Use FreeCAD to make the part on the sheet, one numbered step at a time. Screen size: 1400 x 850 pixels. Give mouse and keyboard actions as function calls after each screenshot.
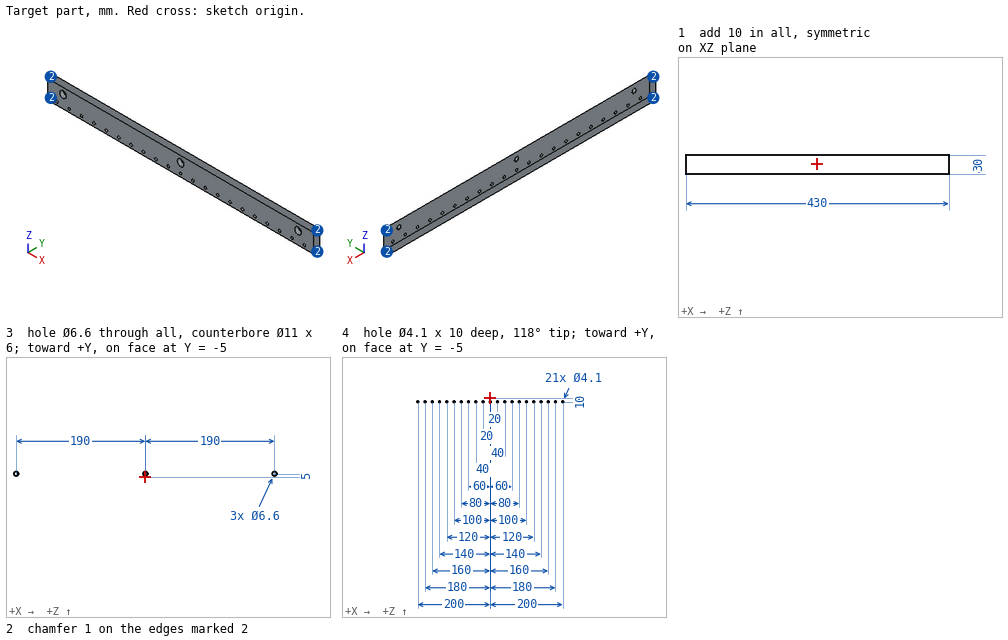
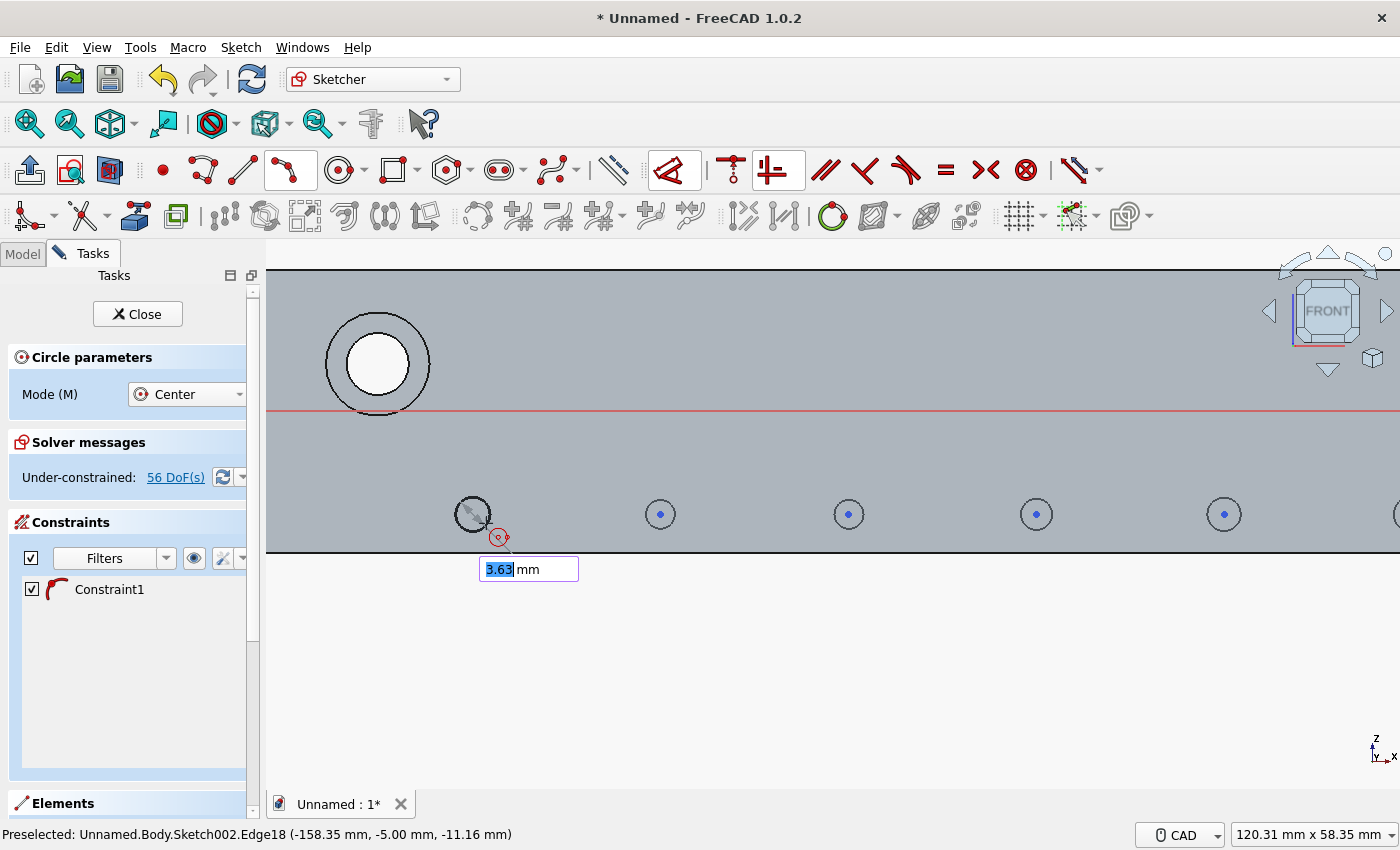
click(486, 519)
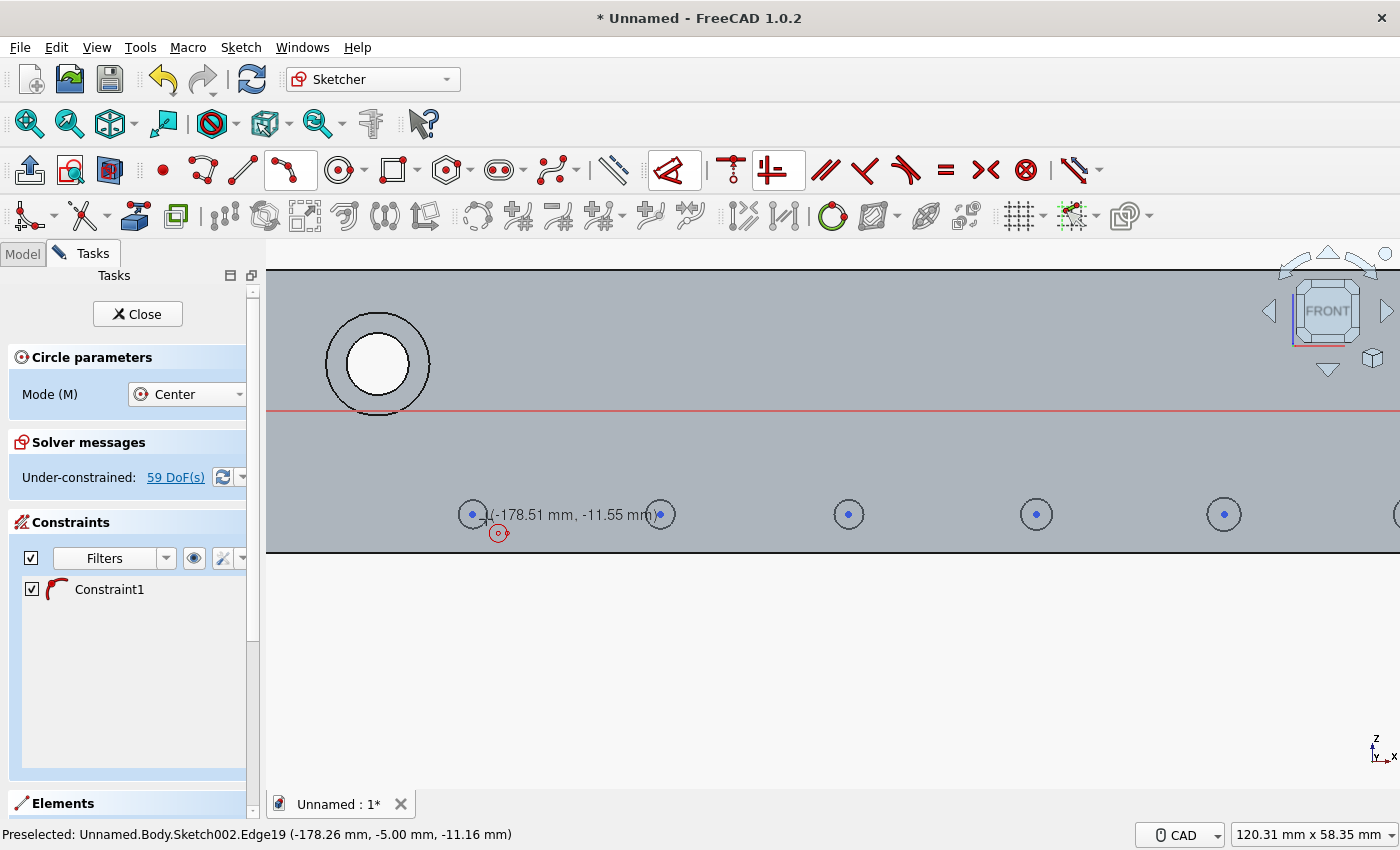
scroll(486, 523, down, 9)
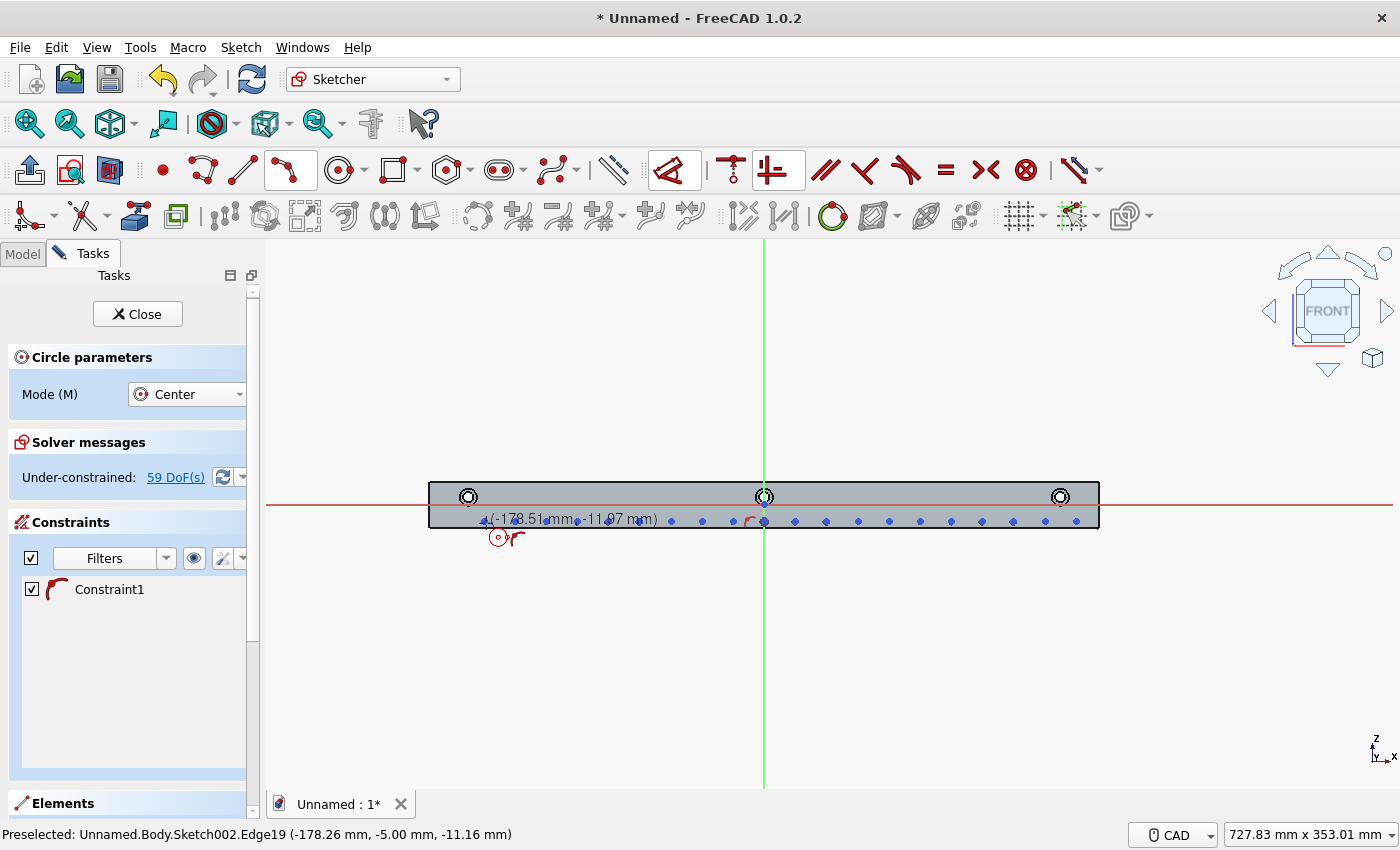
scroll(453, 521, up, 10)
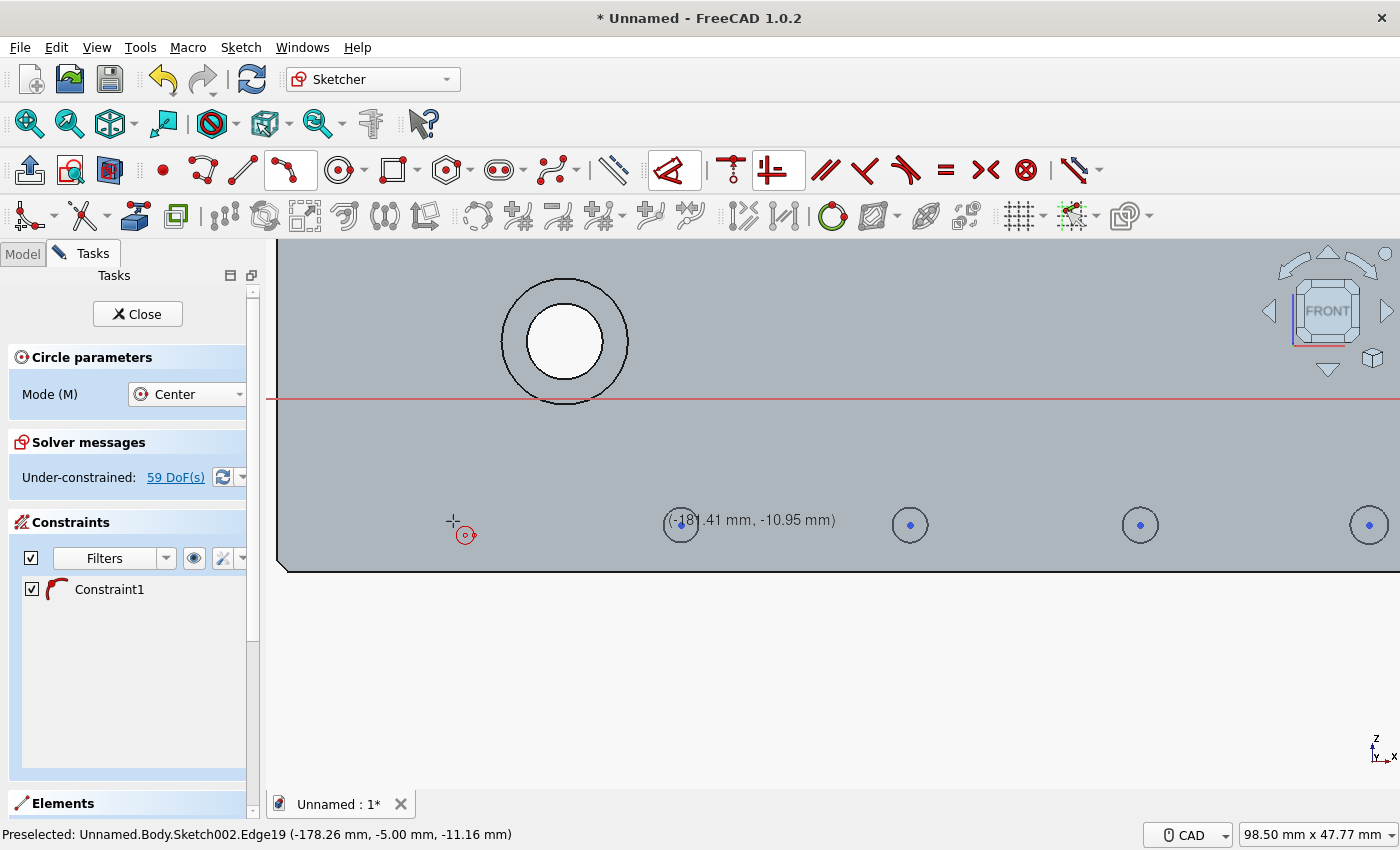
scroll(453, 521, down, 10)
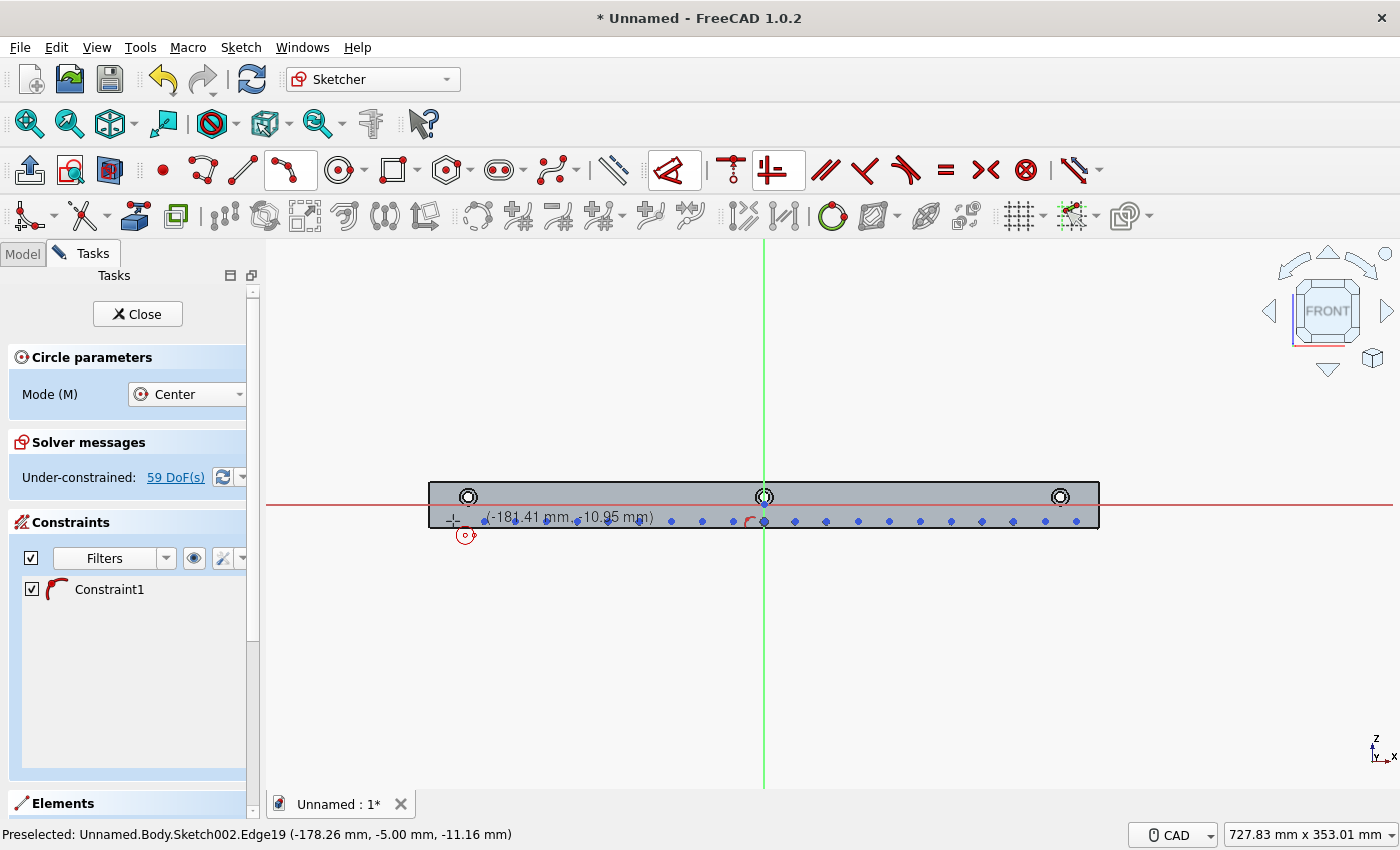
click(453, 521)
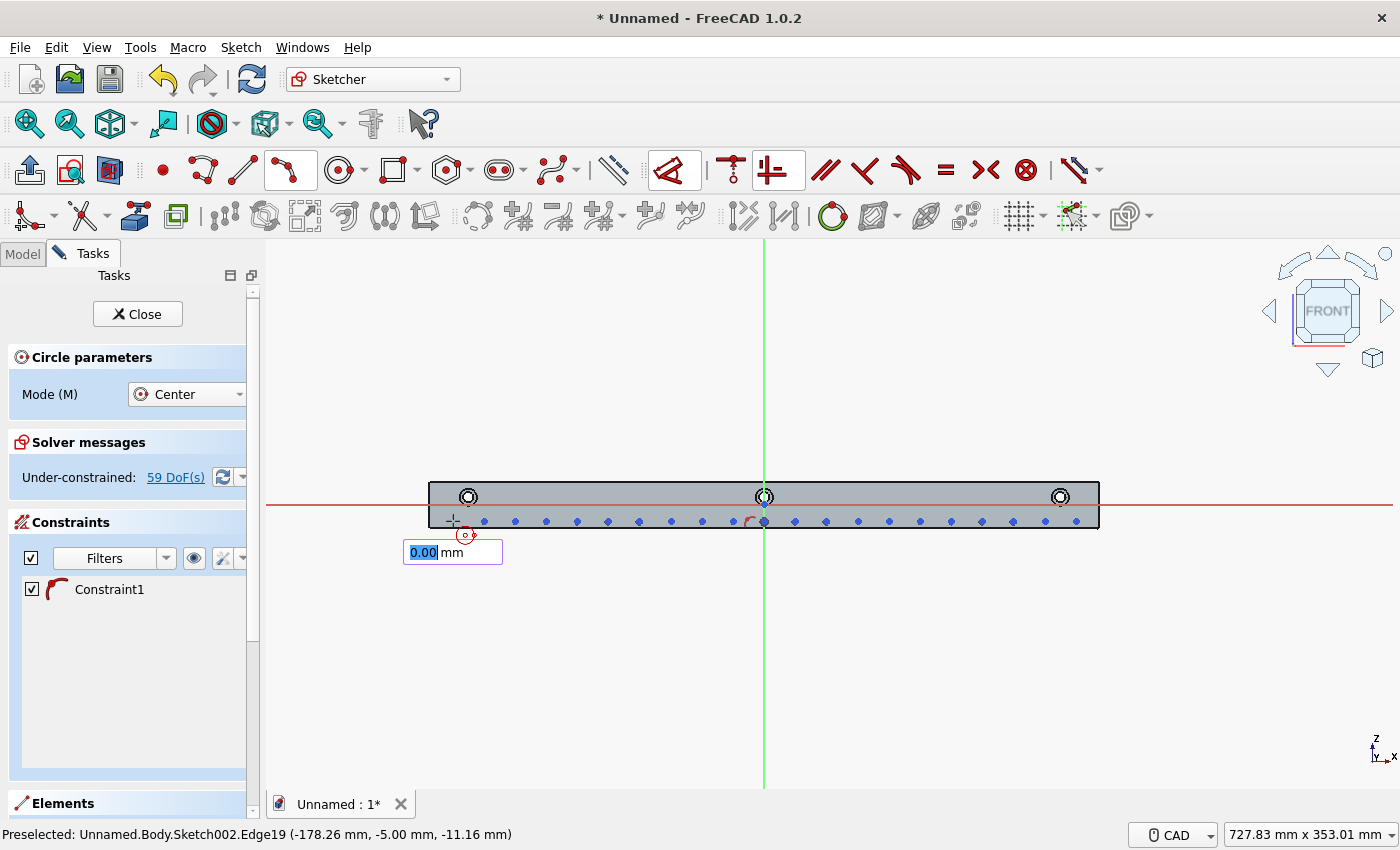
scroll(455, 523, up, 9)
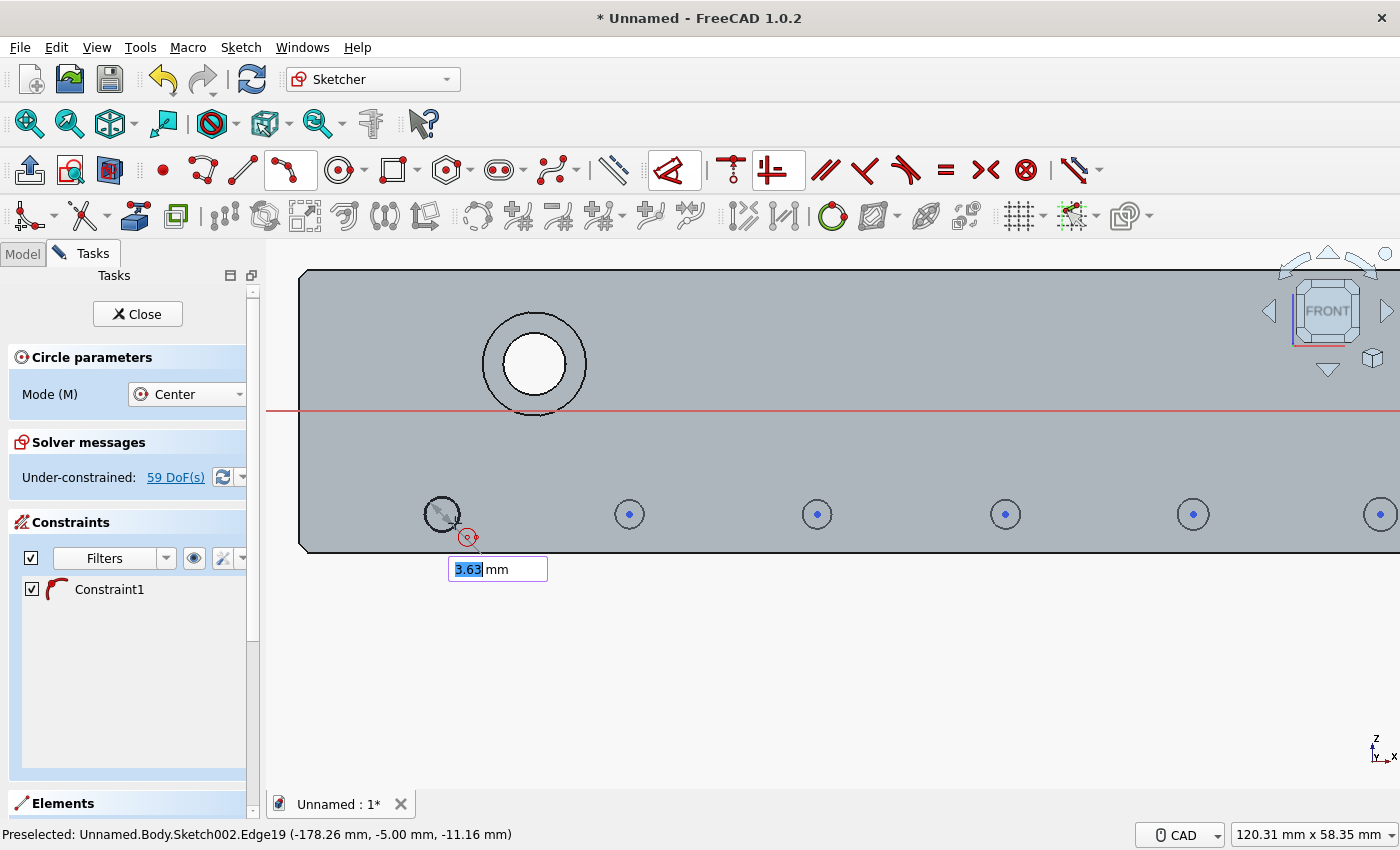
click(454, 519)
key(Escape)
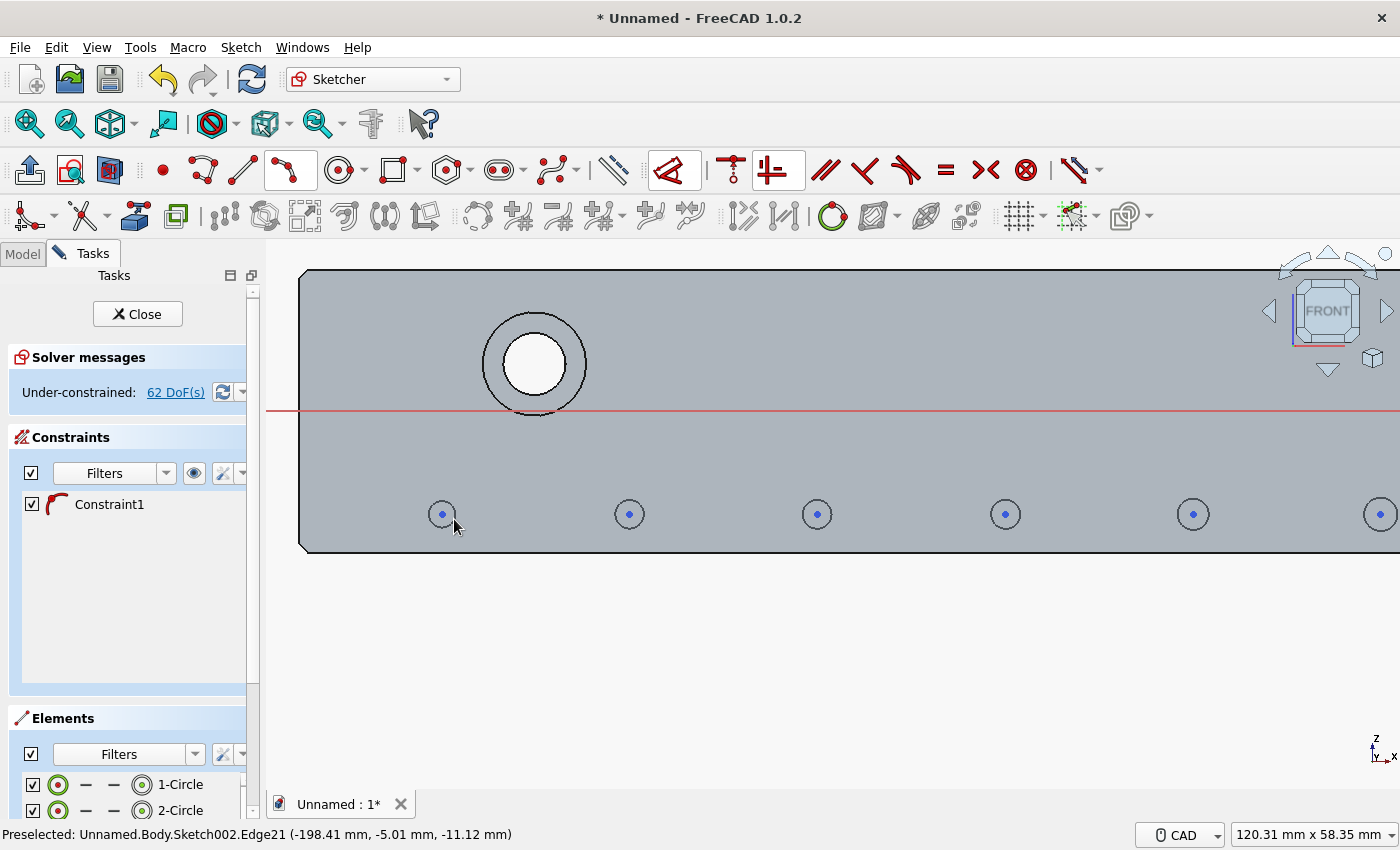
scroll(455, 523, down, 9)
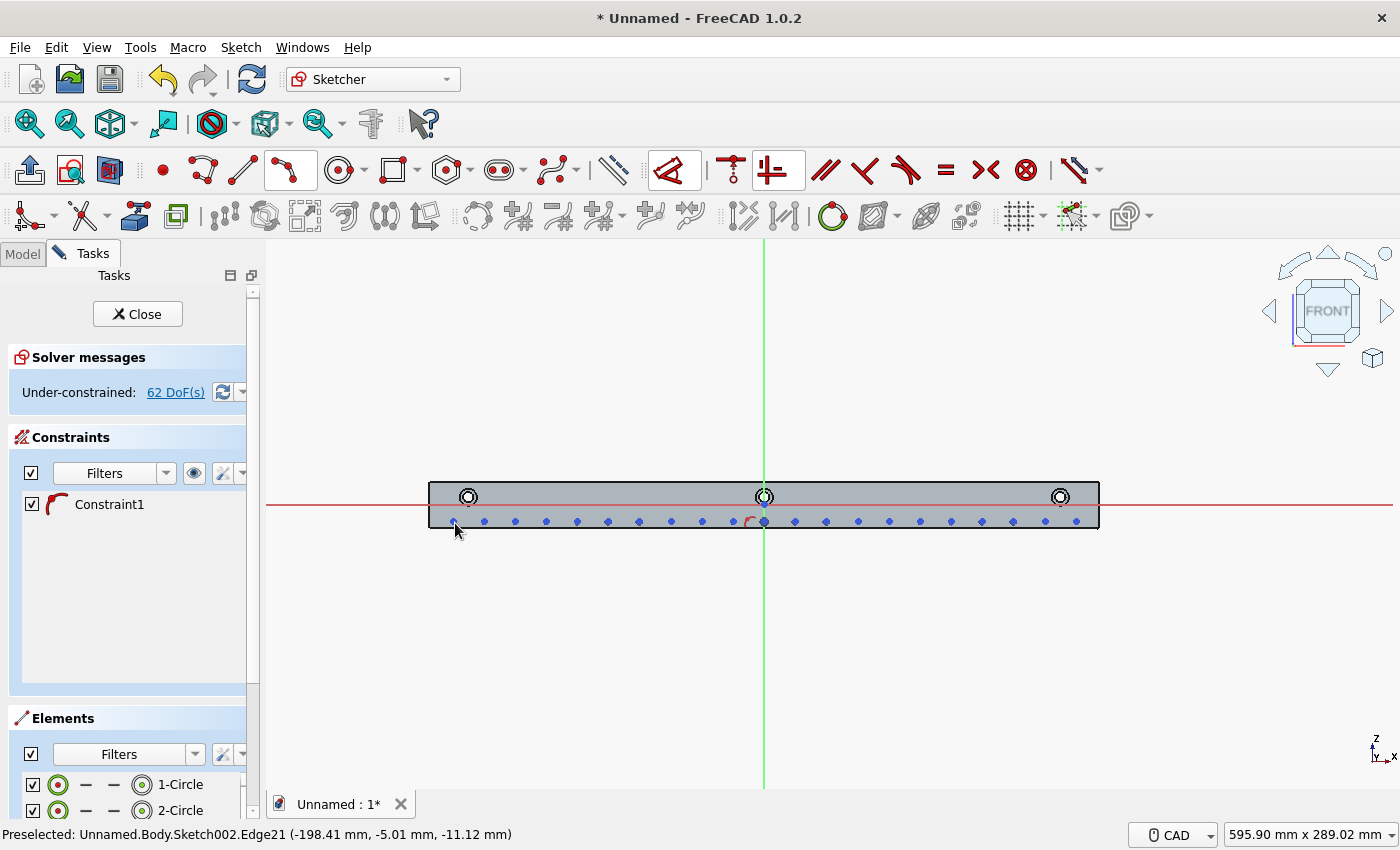
scroll(1078, 520, up, 10)